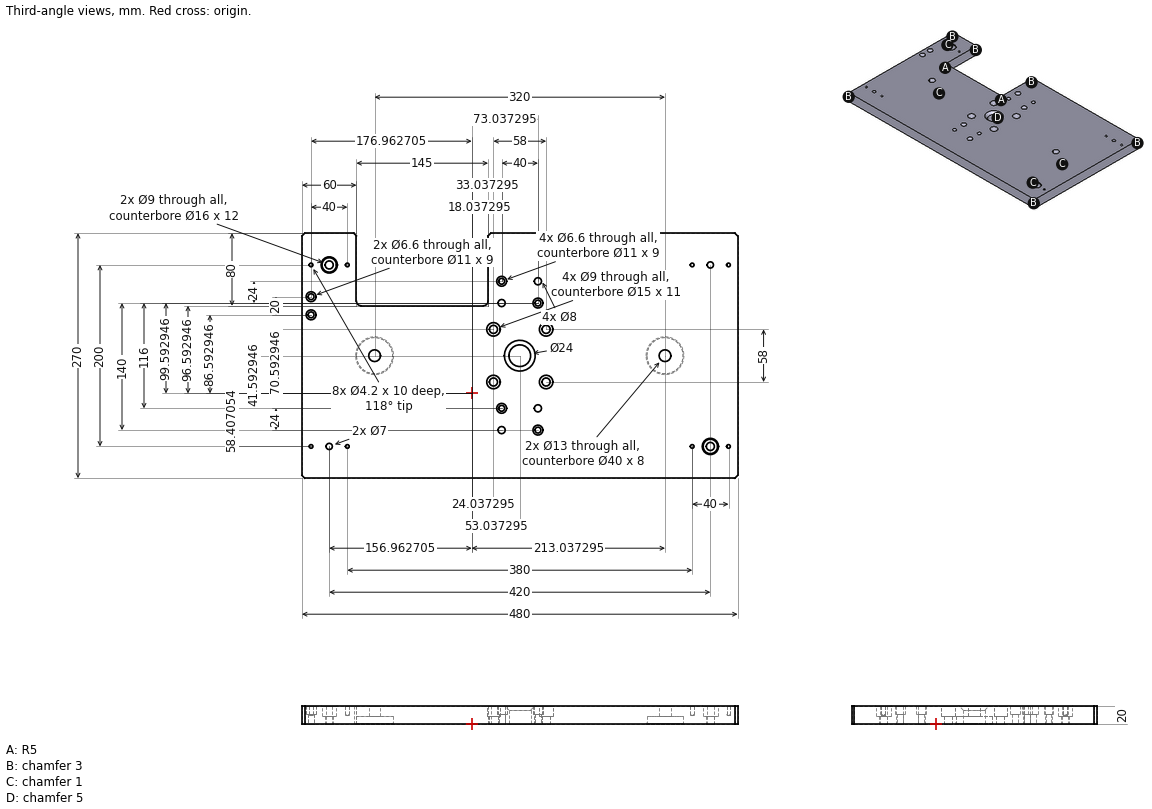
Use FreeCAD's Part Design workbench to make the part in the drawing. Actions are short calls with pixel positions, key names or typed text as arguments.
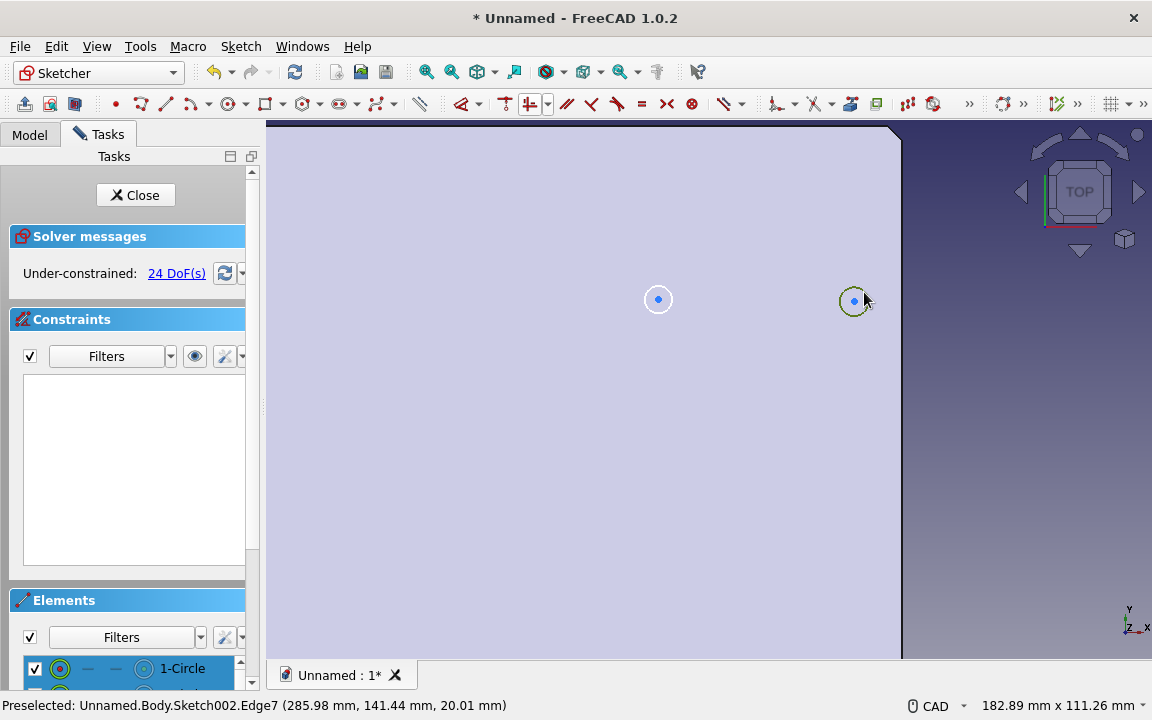
click(668, 290)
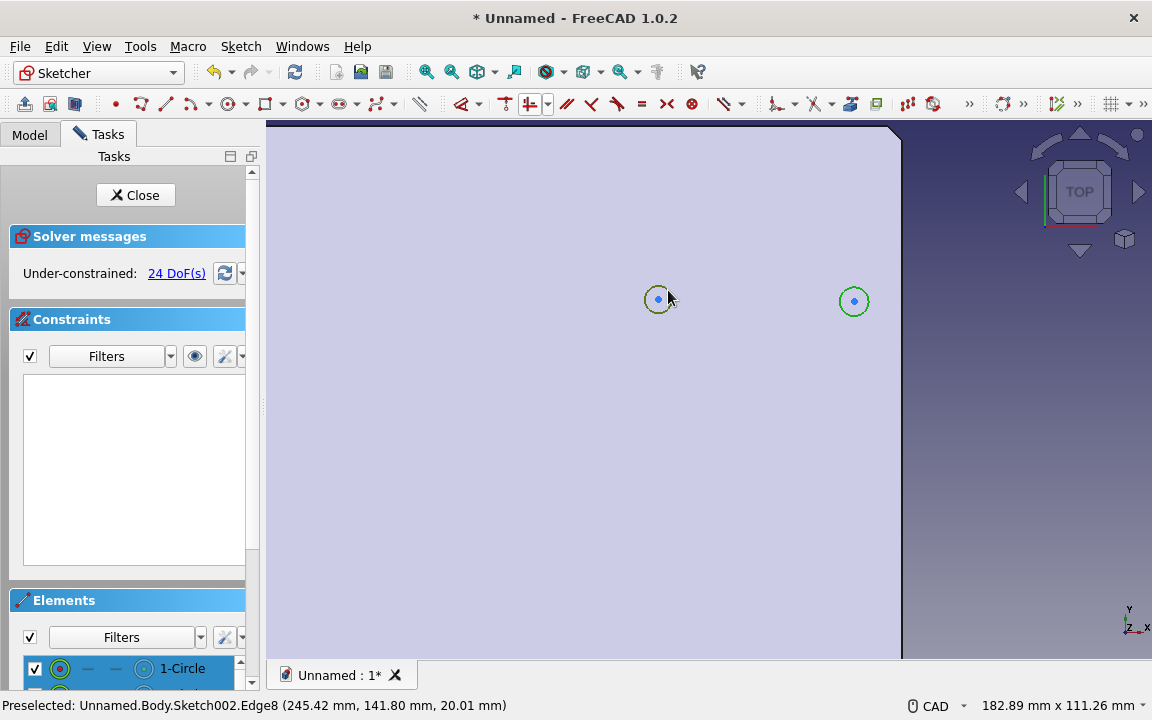
click(642, 104)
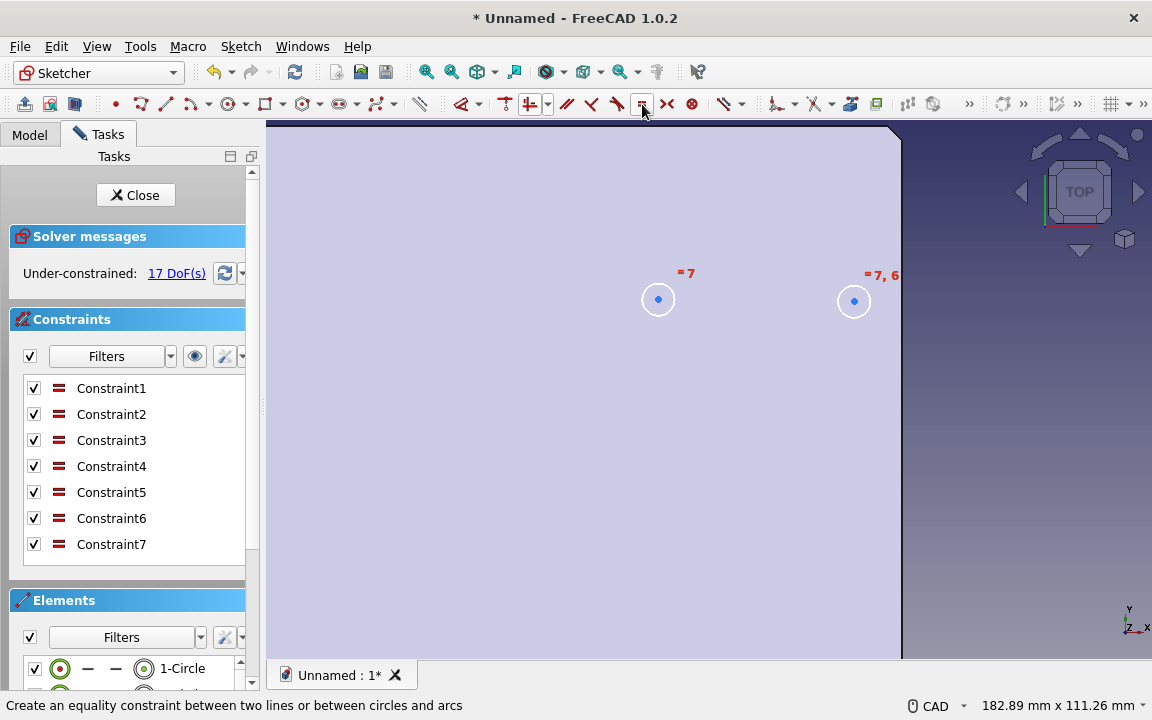
scroll(869, 291, down, 8)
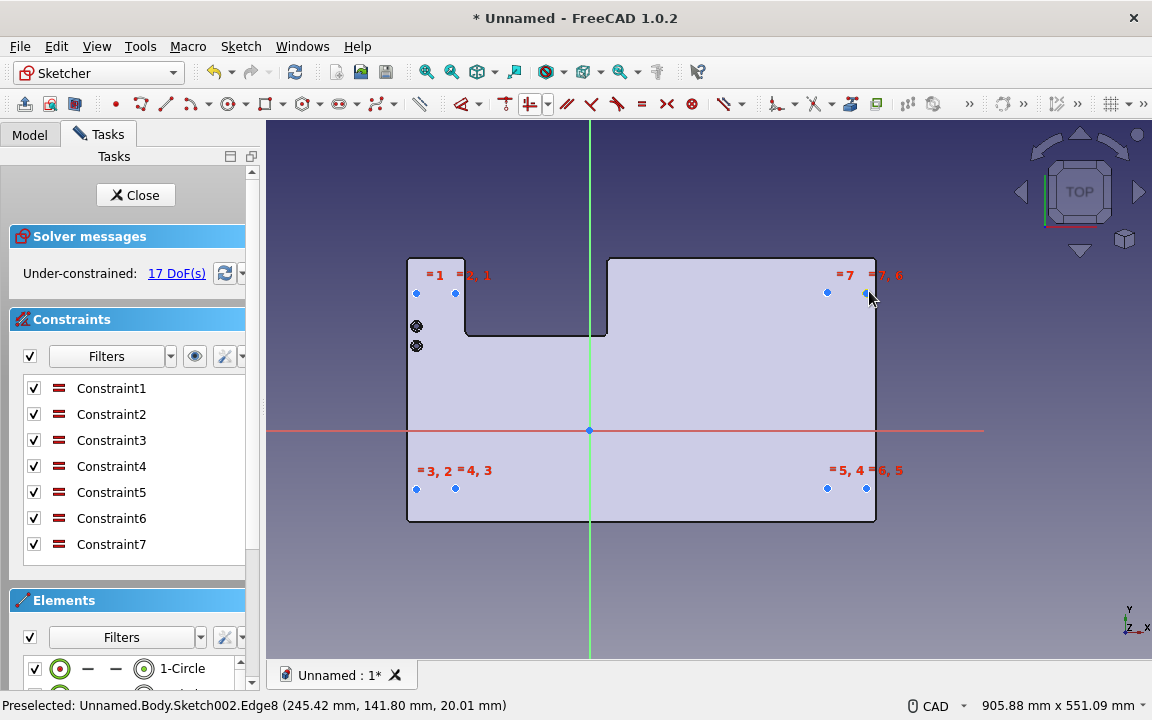
click(416, 294)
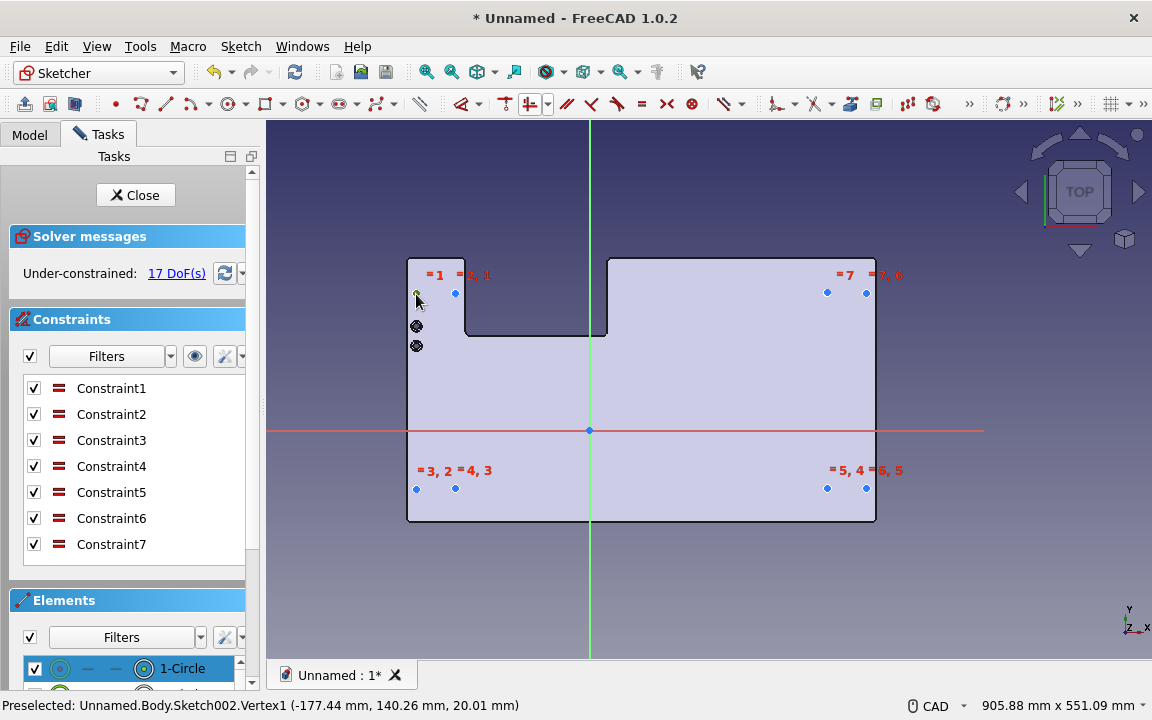
click(455, 293)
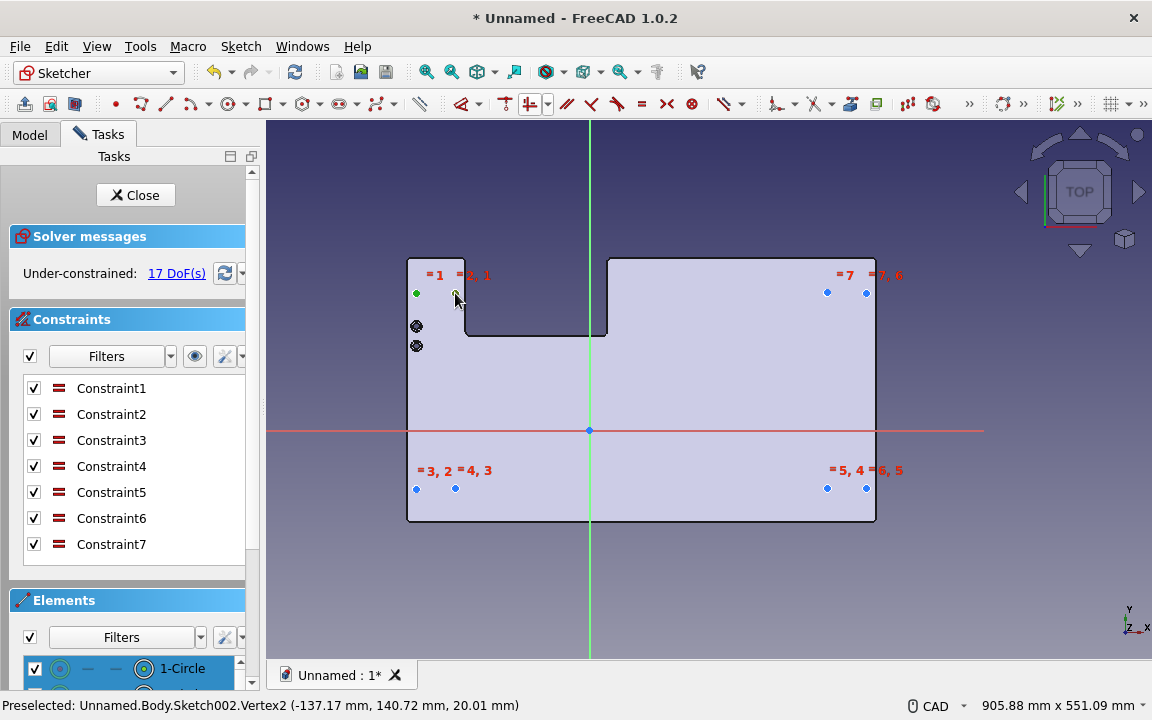
key(h)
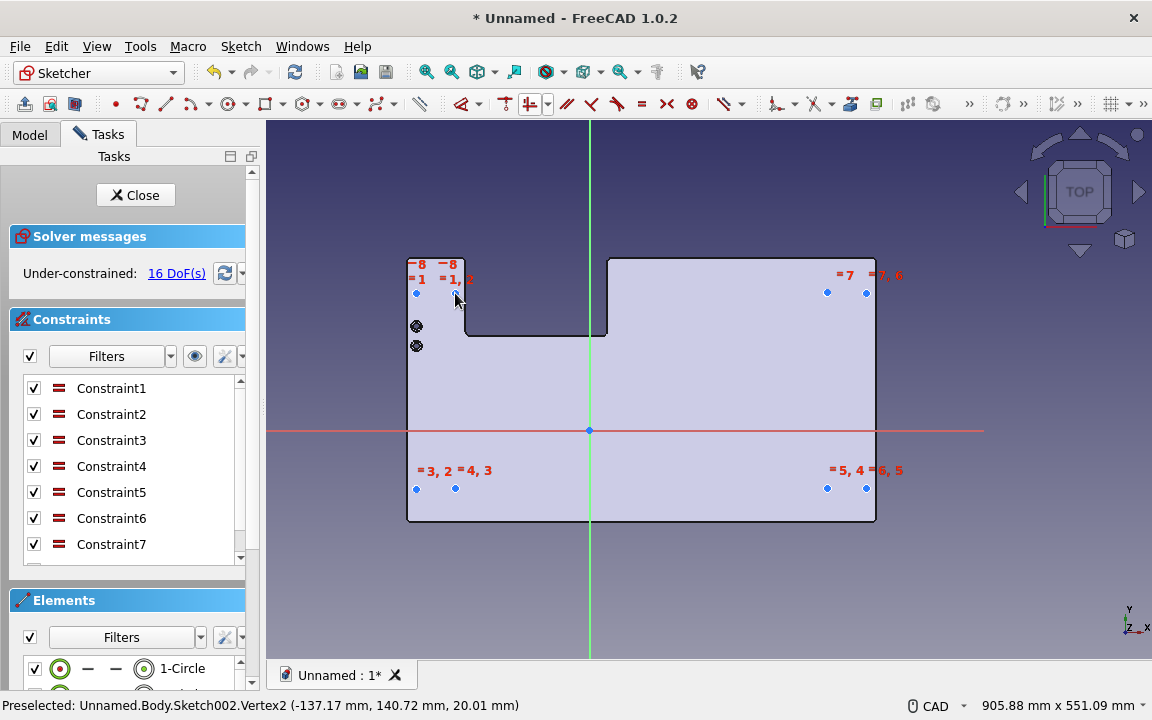
click(416, 294)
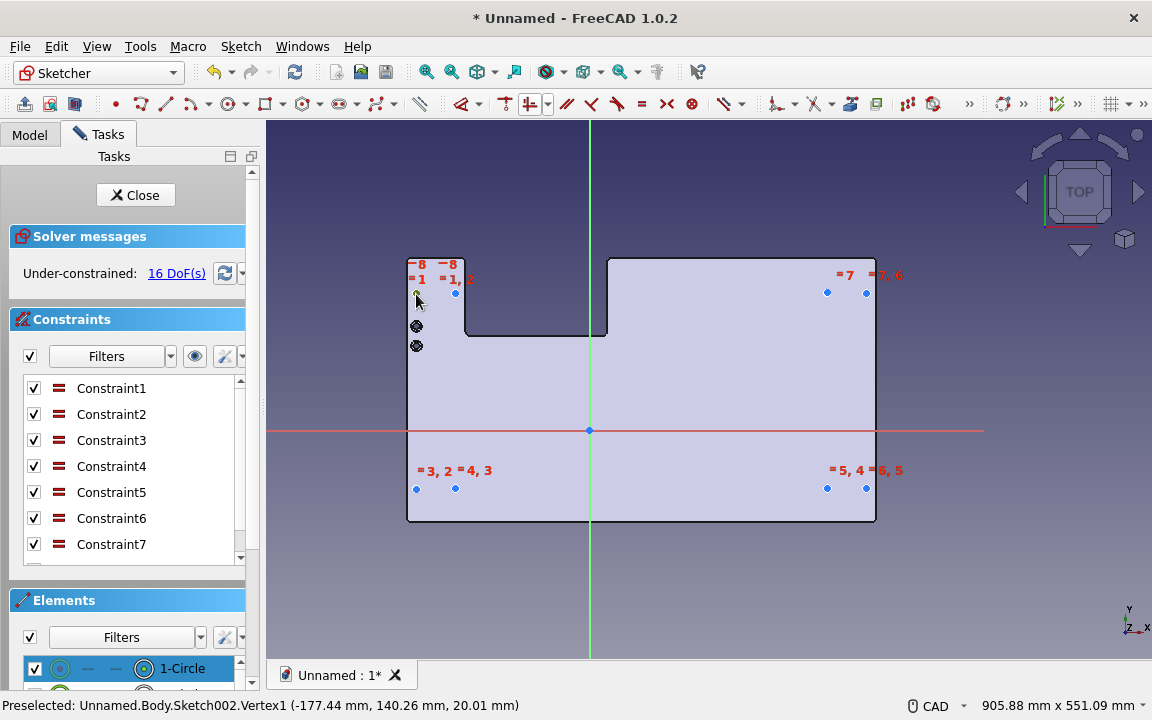
click(416, 489)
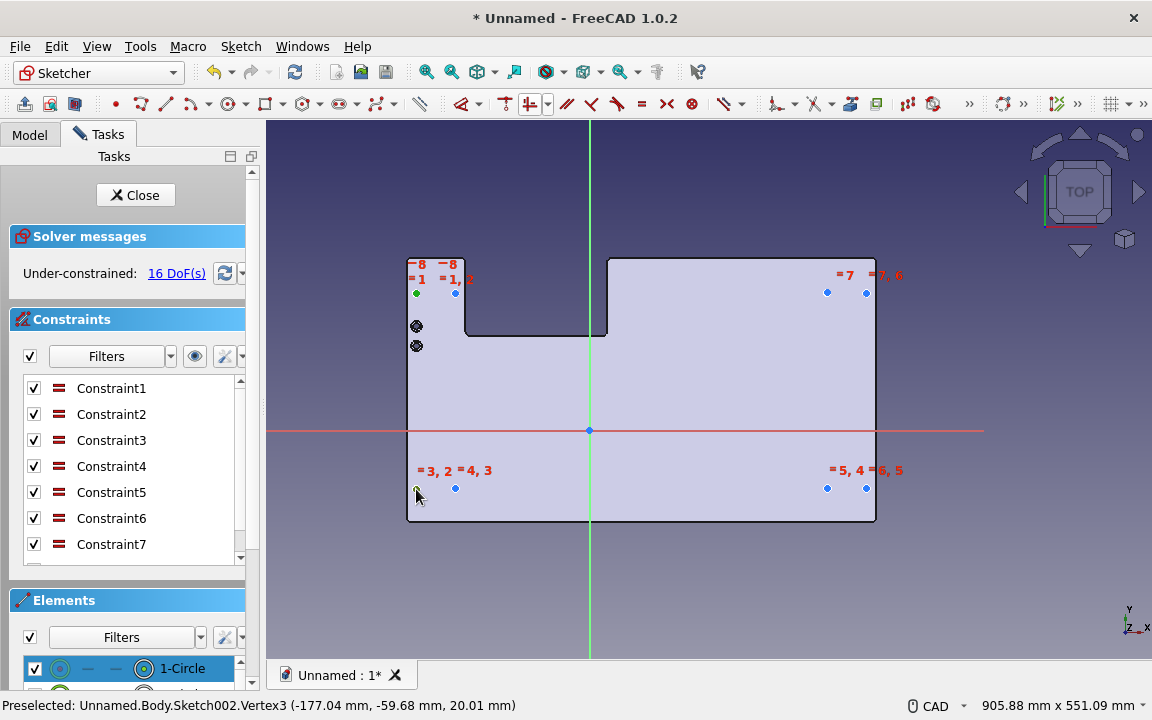
key(v)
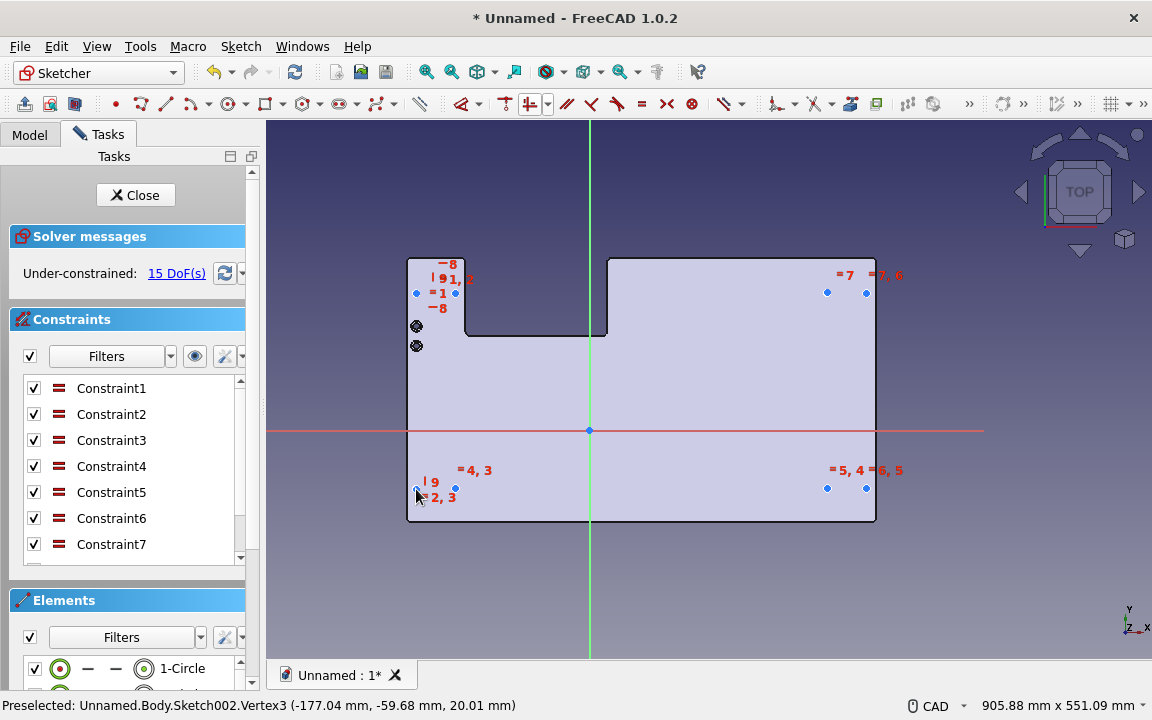
click(455, 294)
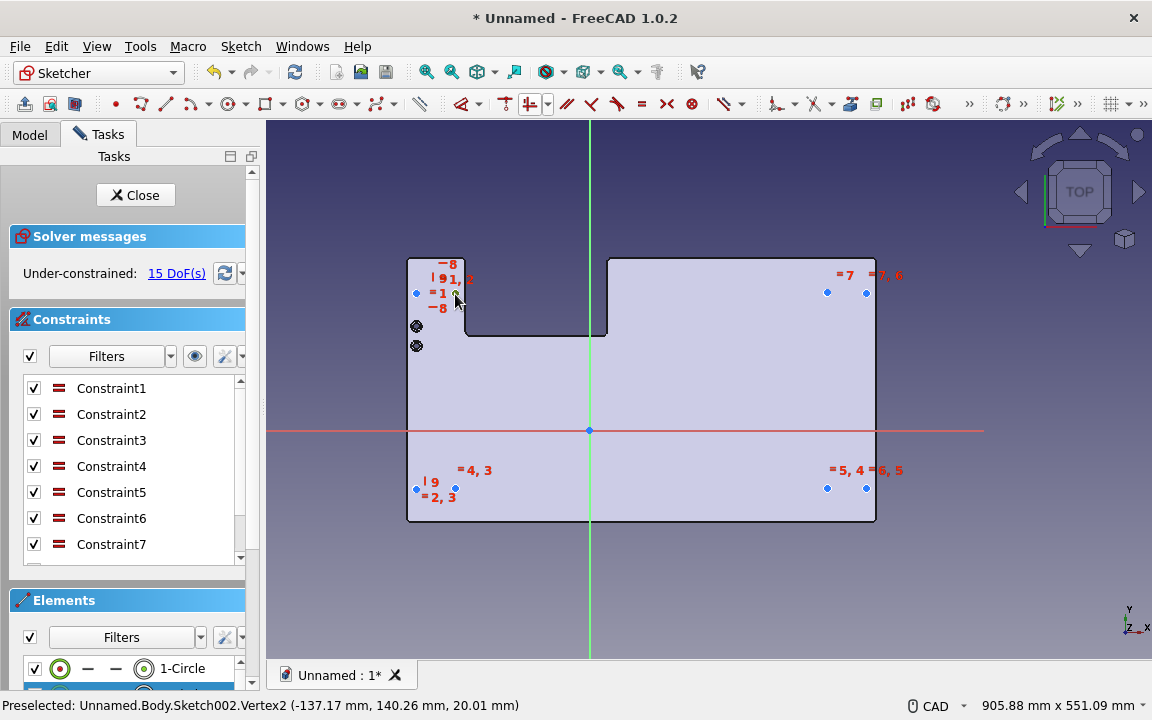
click(458, 490)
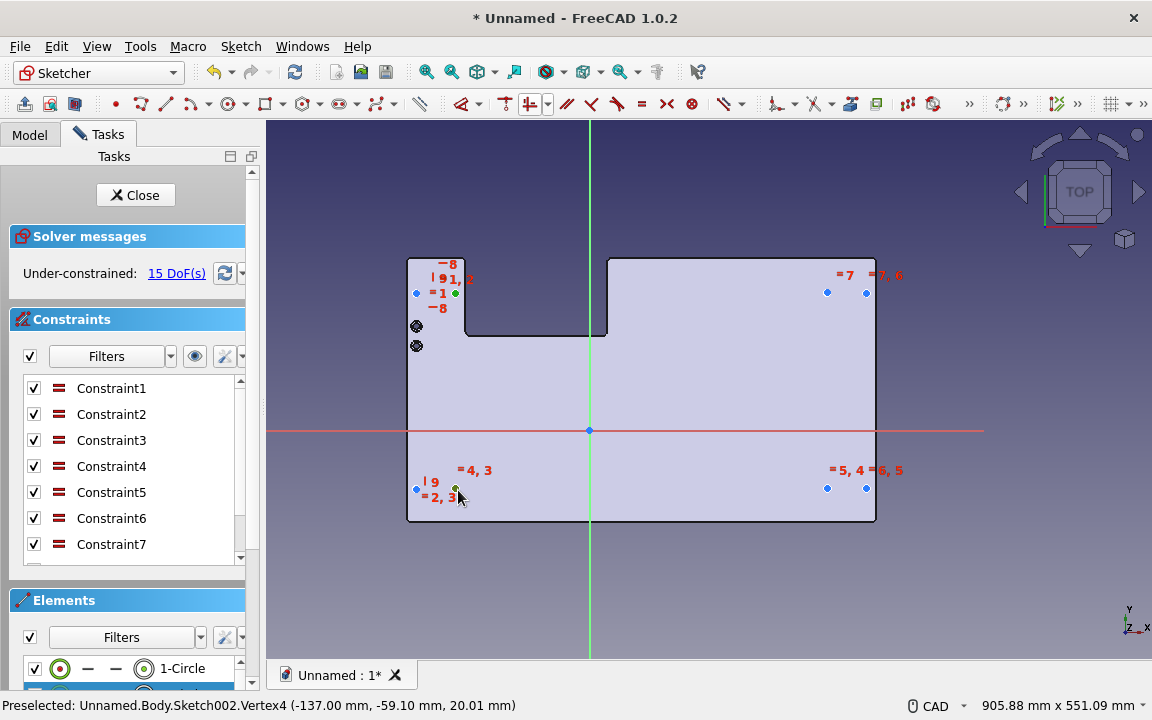
key(v)